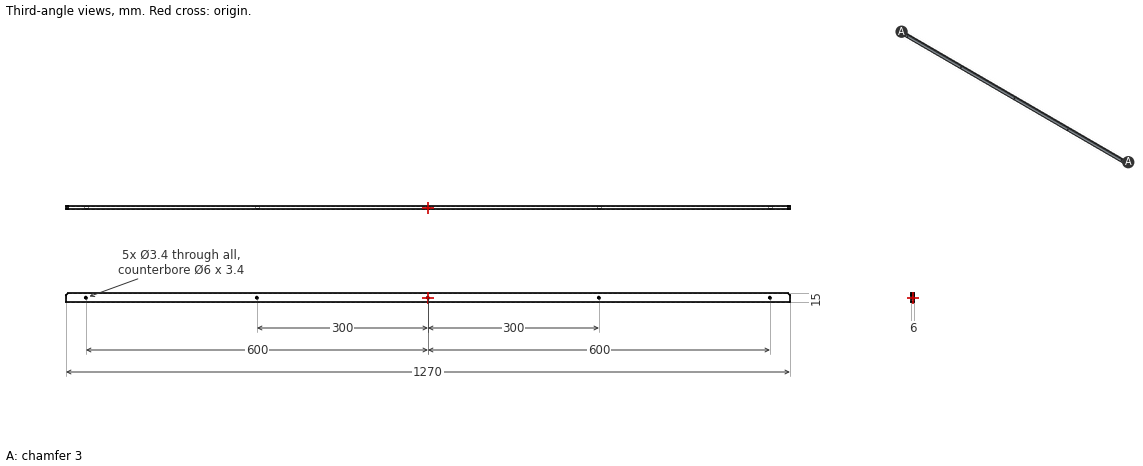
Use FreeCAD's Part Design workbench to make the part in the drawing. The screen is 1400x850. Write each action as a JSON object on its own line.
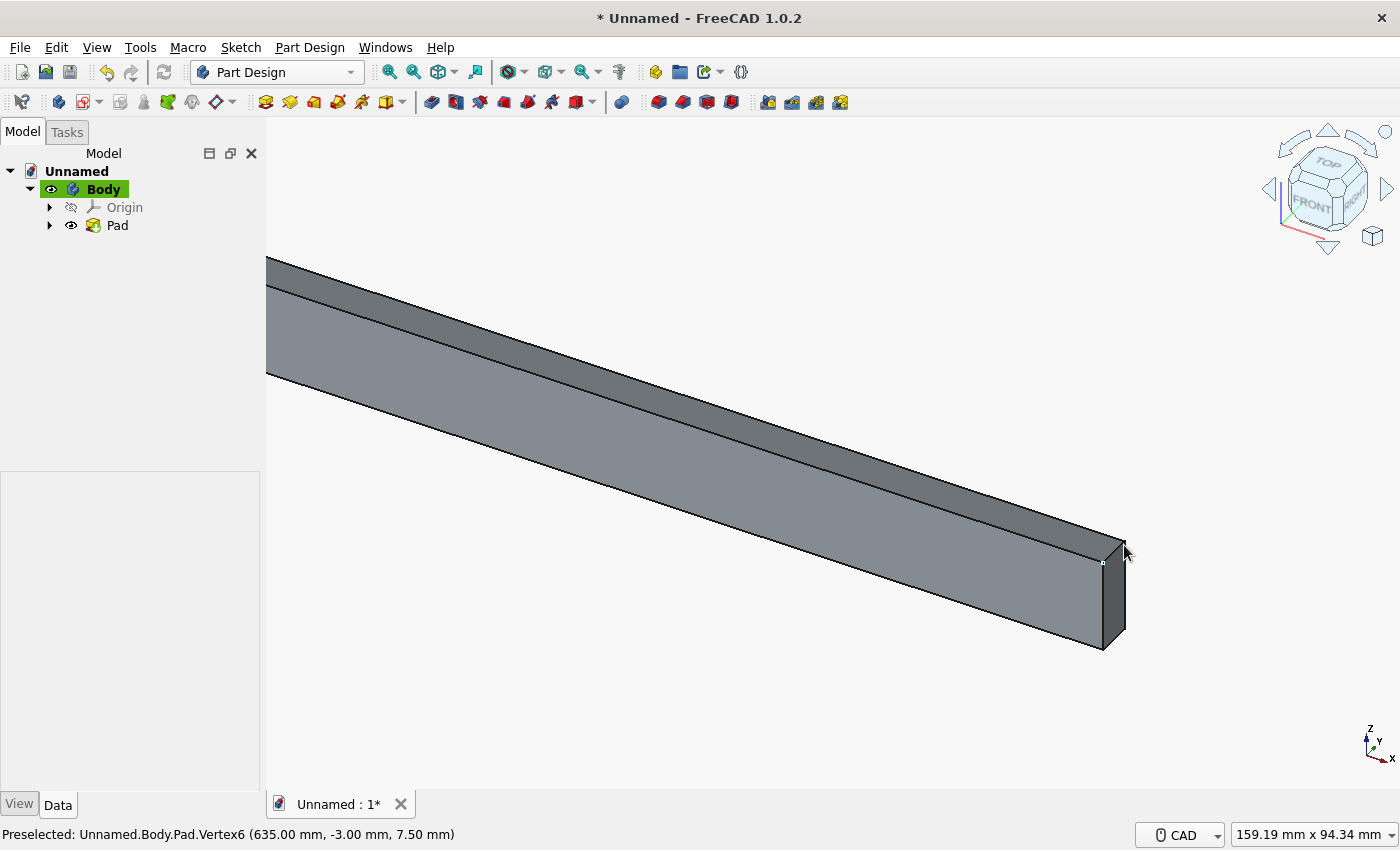
{"action": "left_click", "coordinate": [1114, 551]}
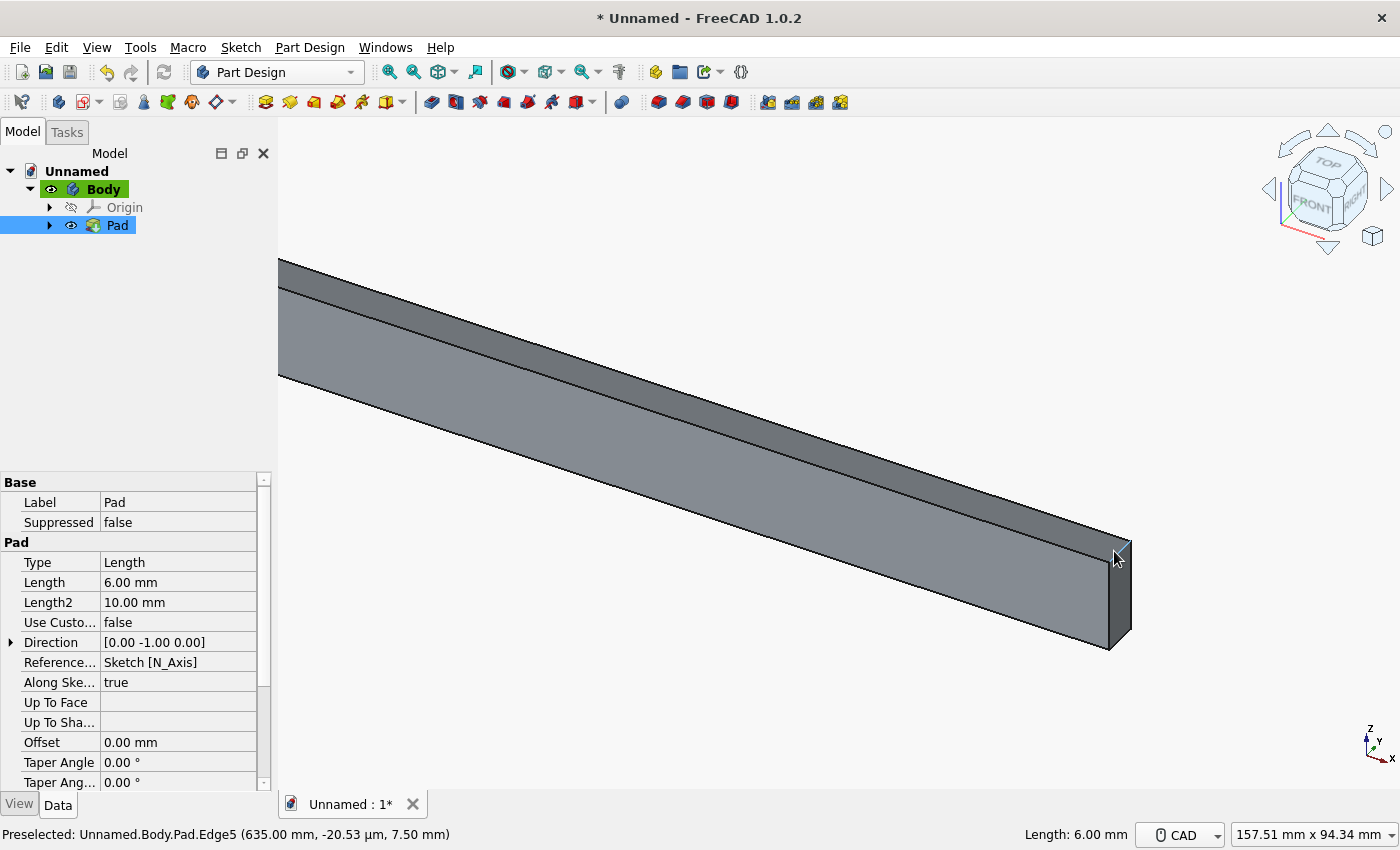
{"action": "key", "text": "v f"}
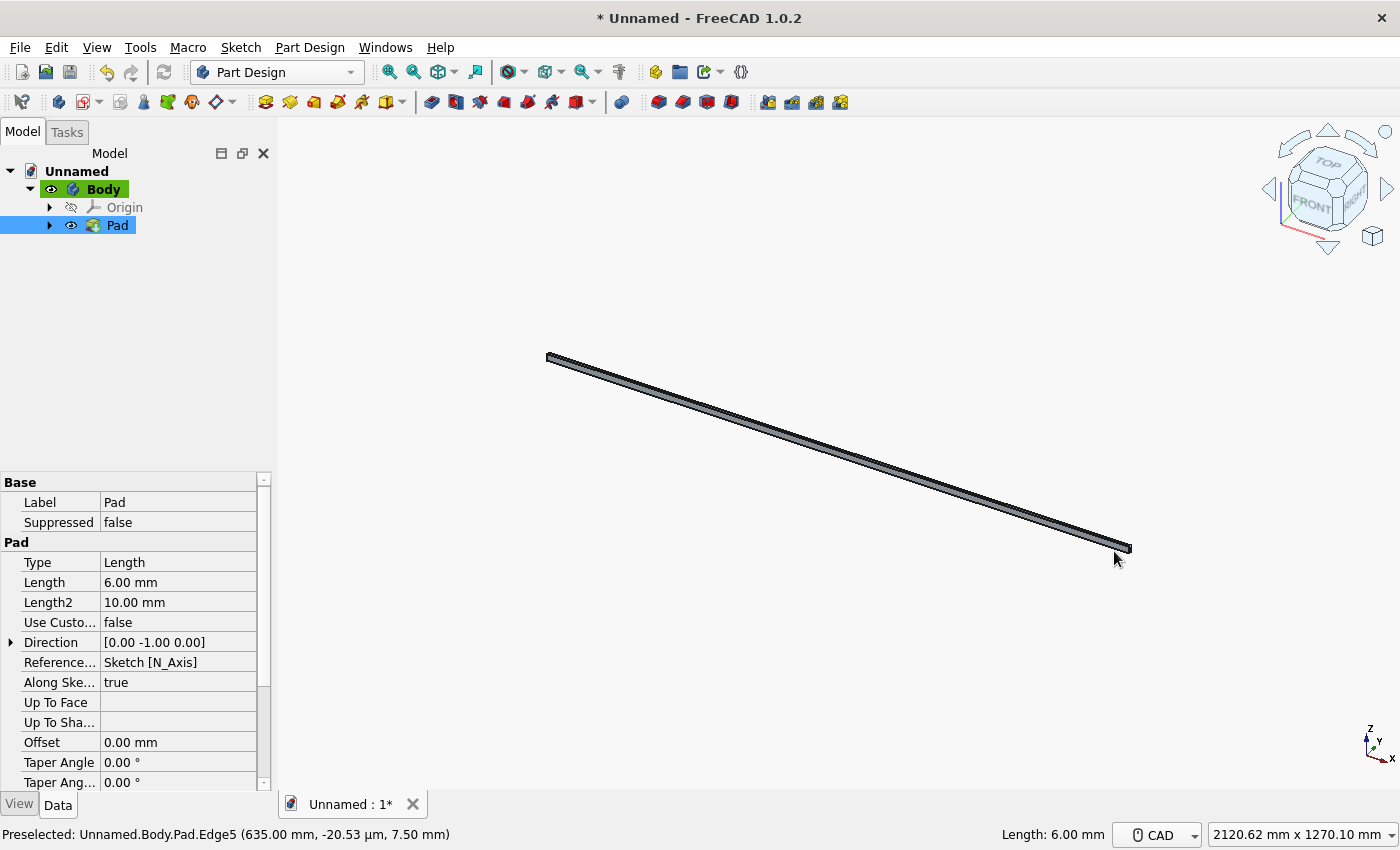
{"action": "key", "text": "0"}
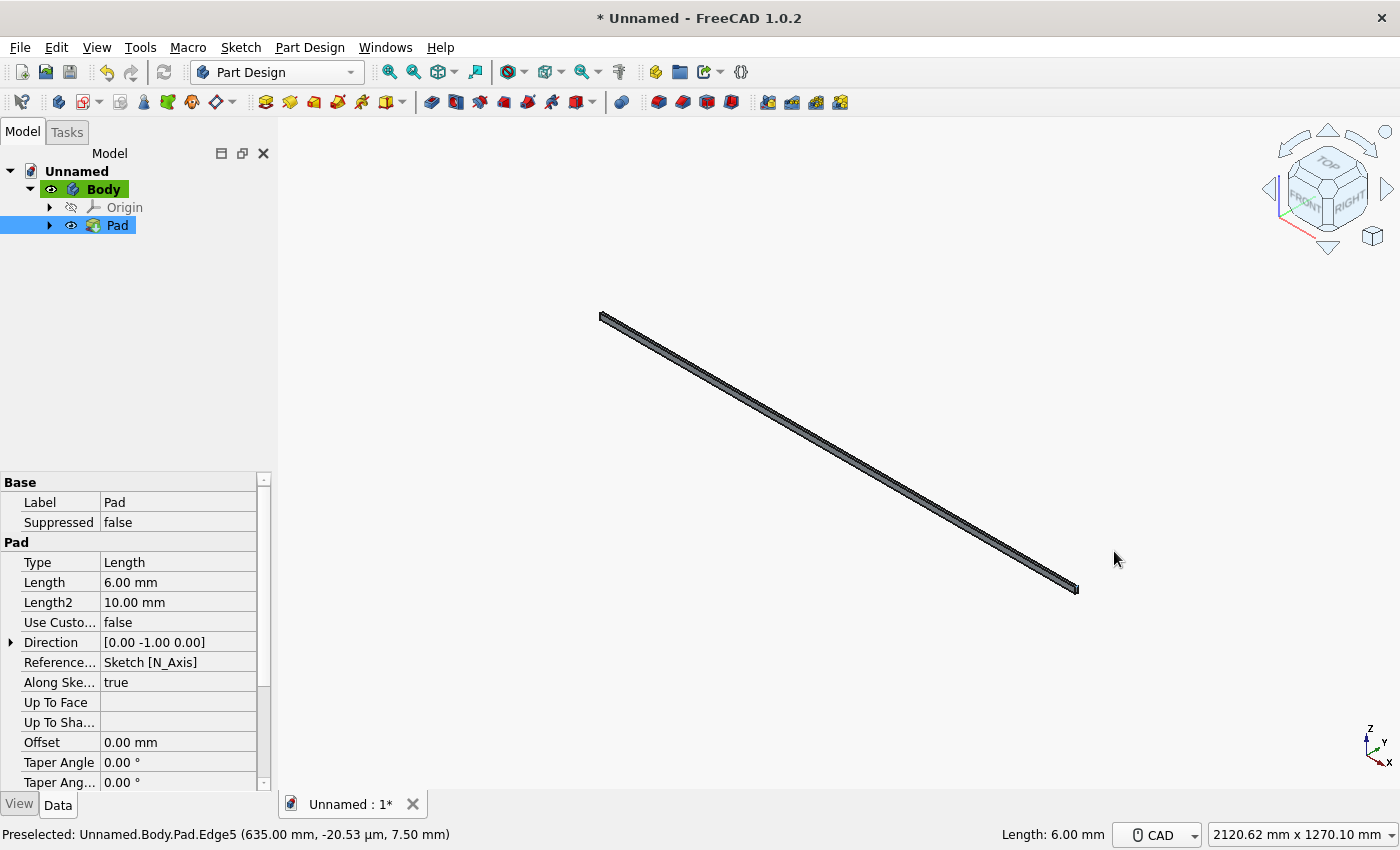
{"action": "key", "text": "v f"}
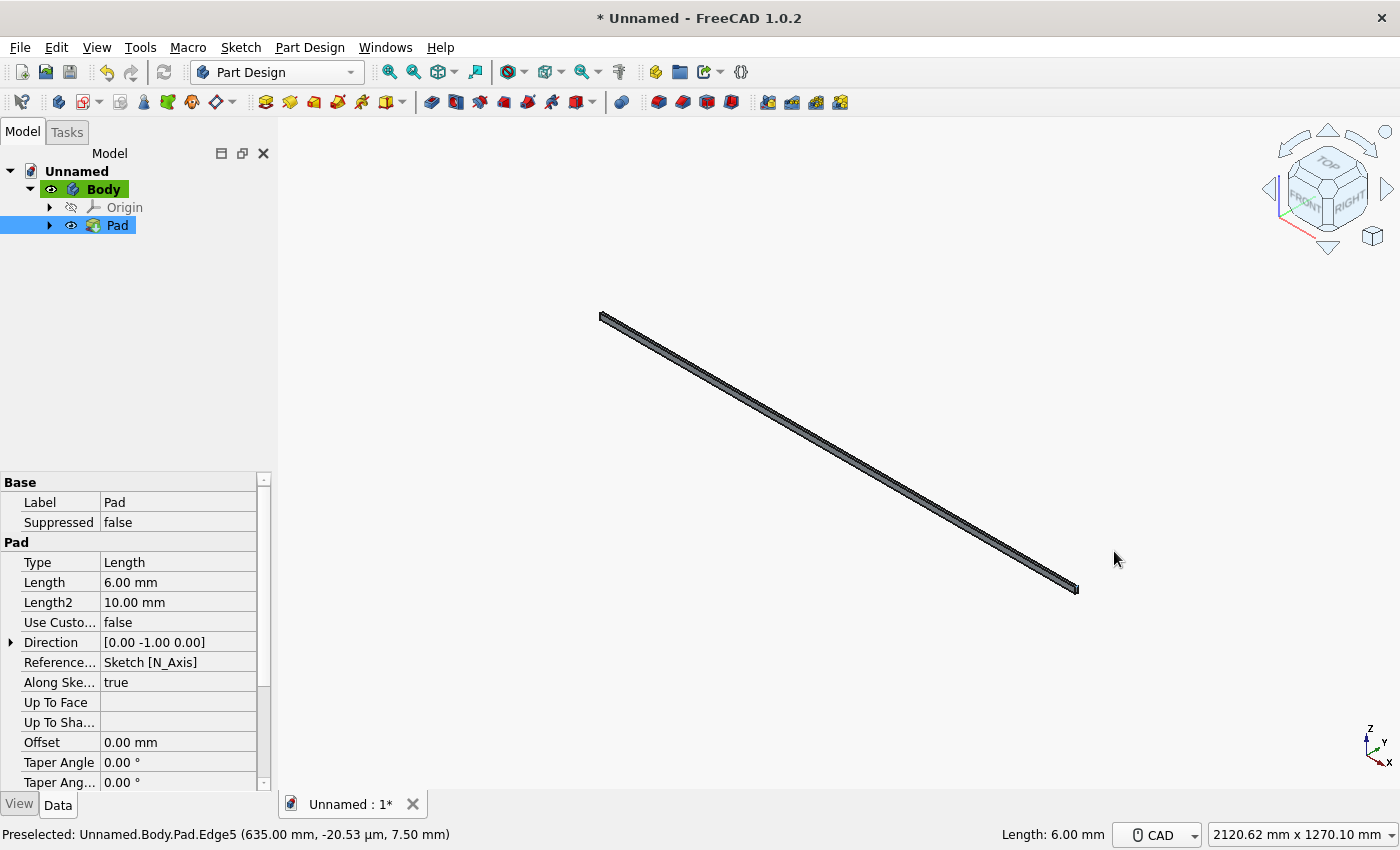
{"action": "scroll", "coordinate": [601, 312], "scroll_direction": "up", "scroll_amount": 13}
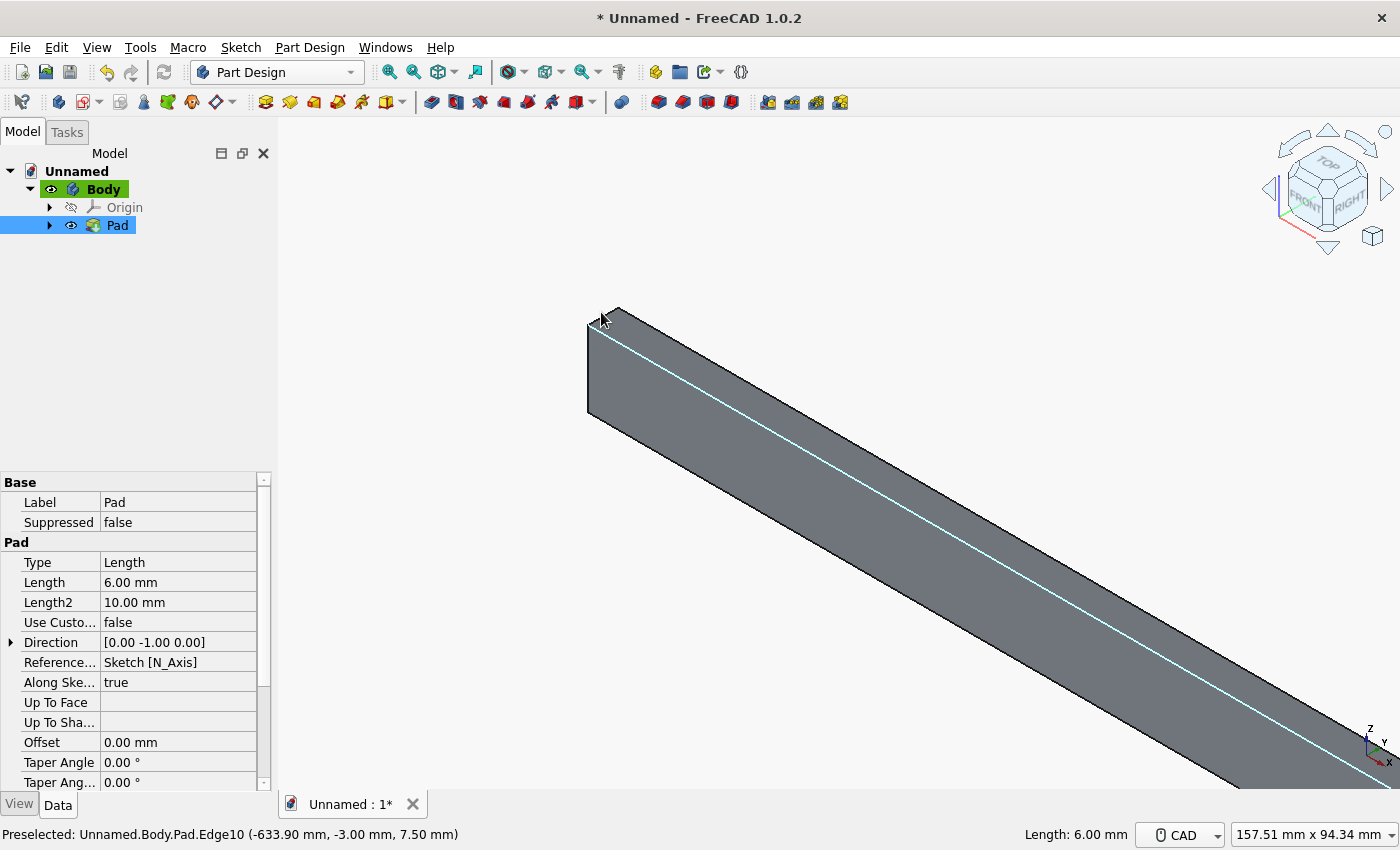
{"action": "left_click", "coordinate": [390, 72]}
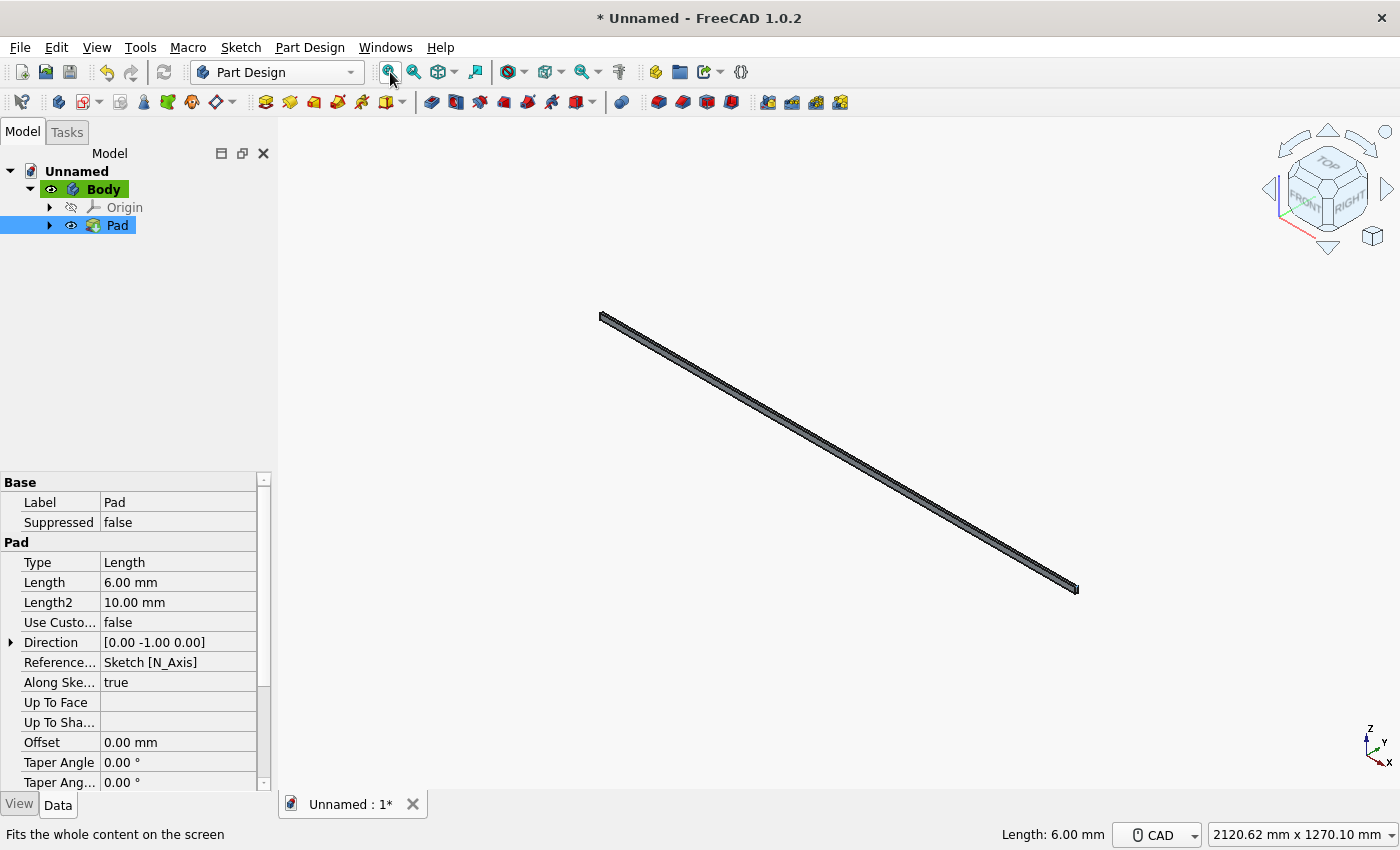
{"action": "key", "text": "2"}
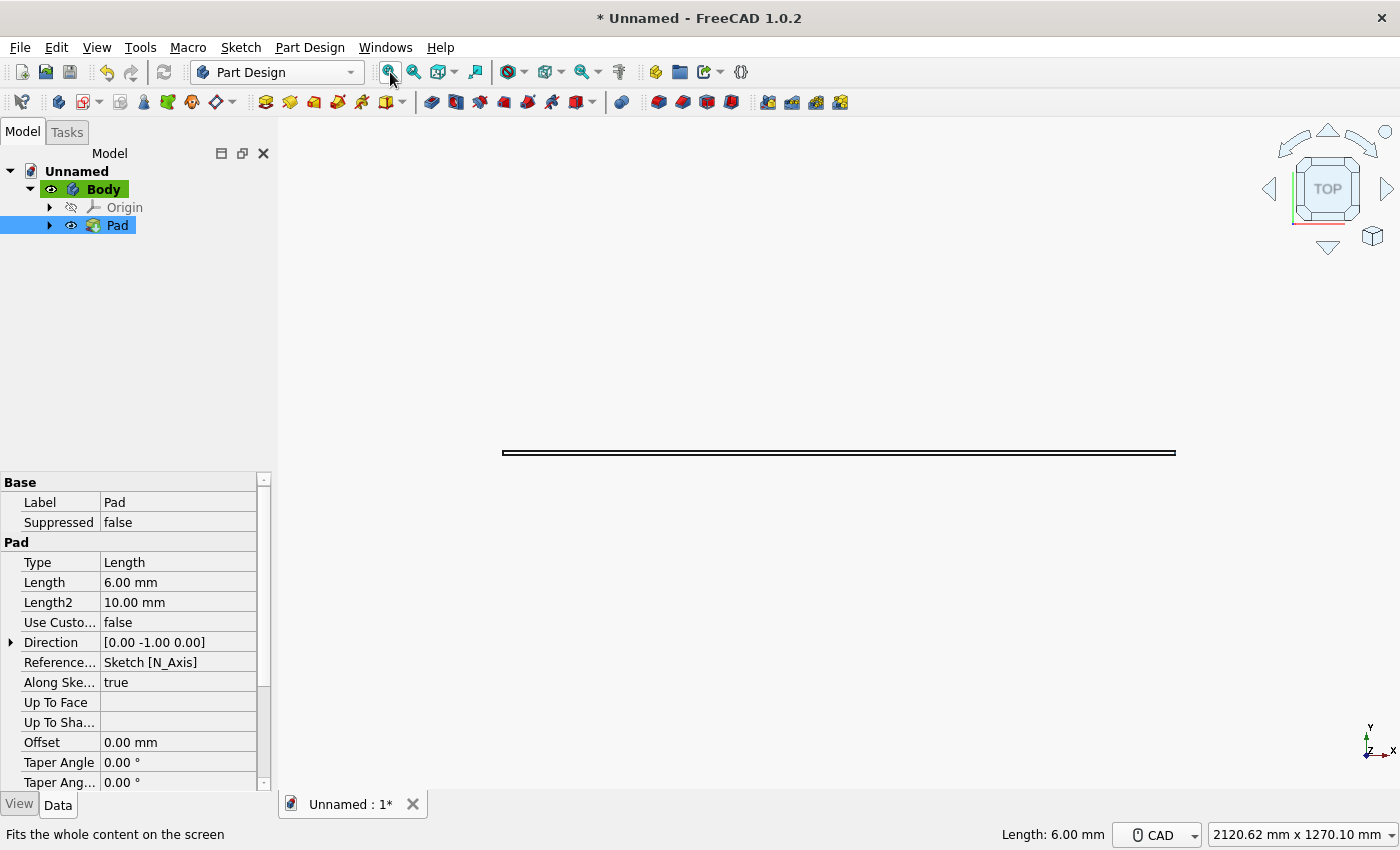
{"action": "scroll", "coordinate": [503, 452], "scroll_direction": "up", "scroll_amount": 13}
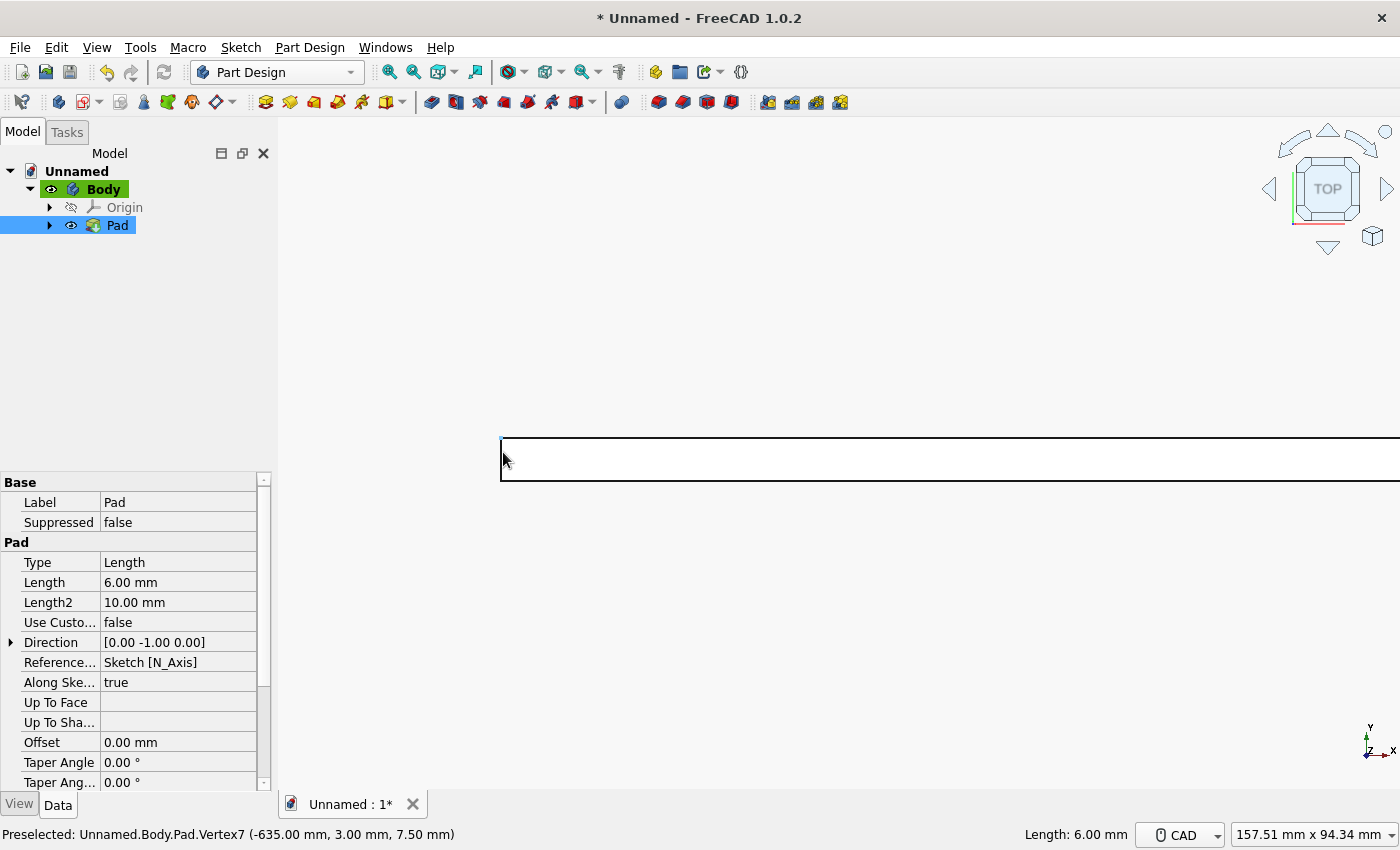
{"action": "left_click", "coordinate": [501, 458], "text": "ctrl"}